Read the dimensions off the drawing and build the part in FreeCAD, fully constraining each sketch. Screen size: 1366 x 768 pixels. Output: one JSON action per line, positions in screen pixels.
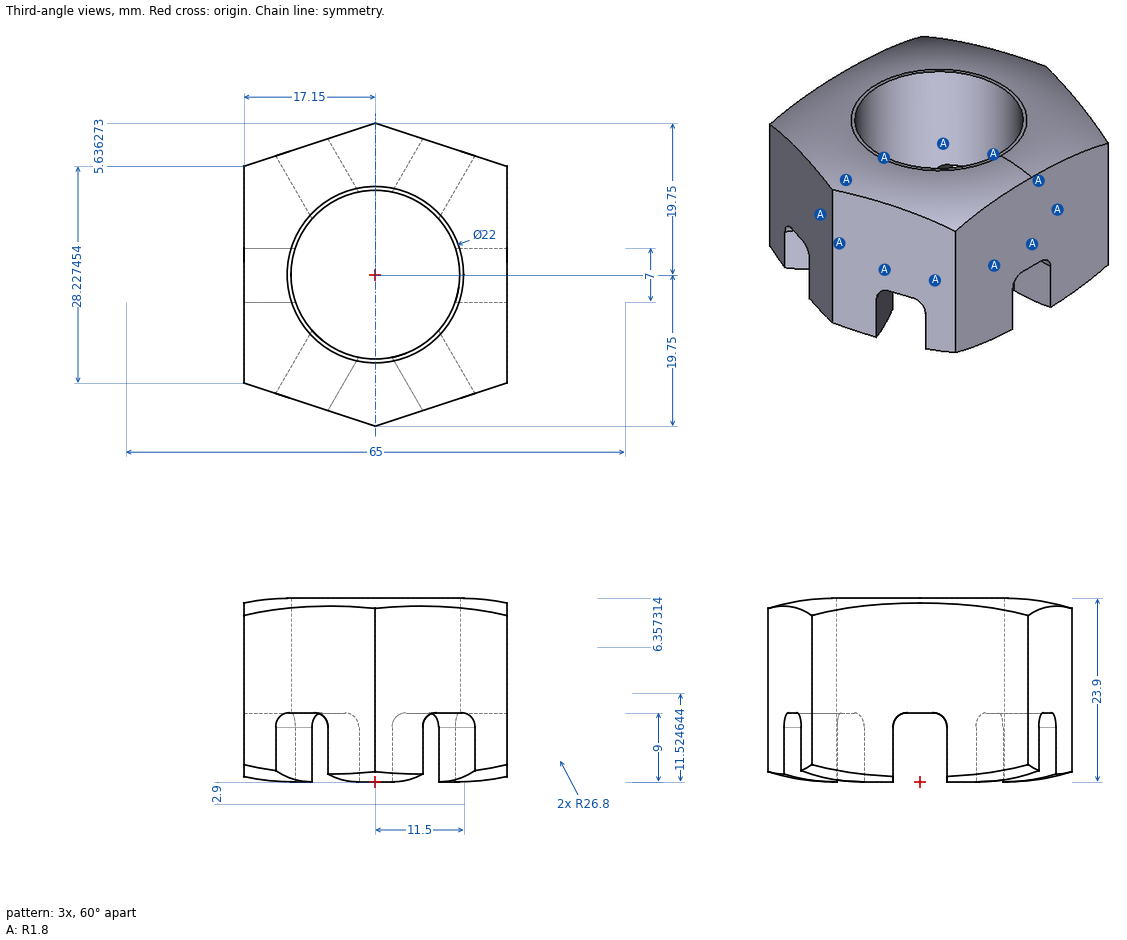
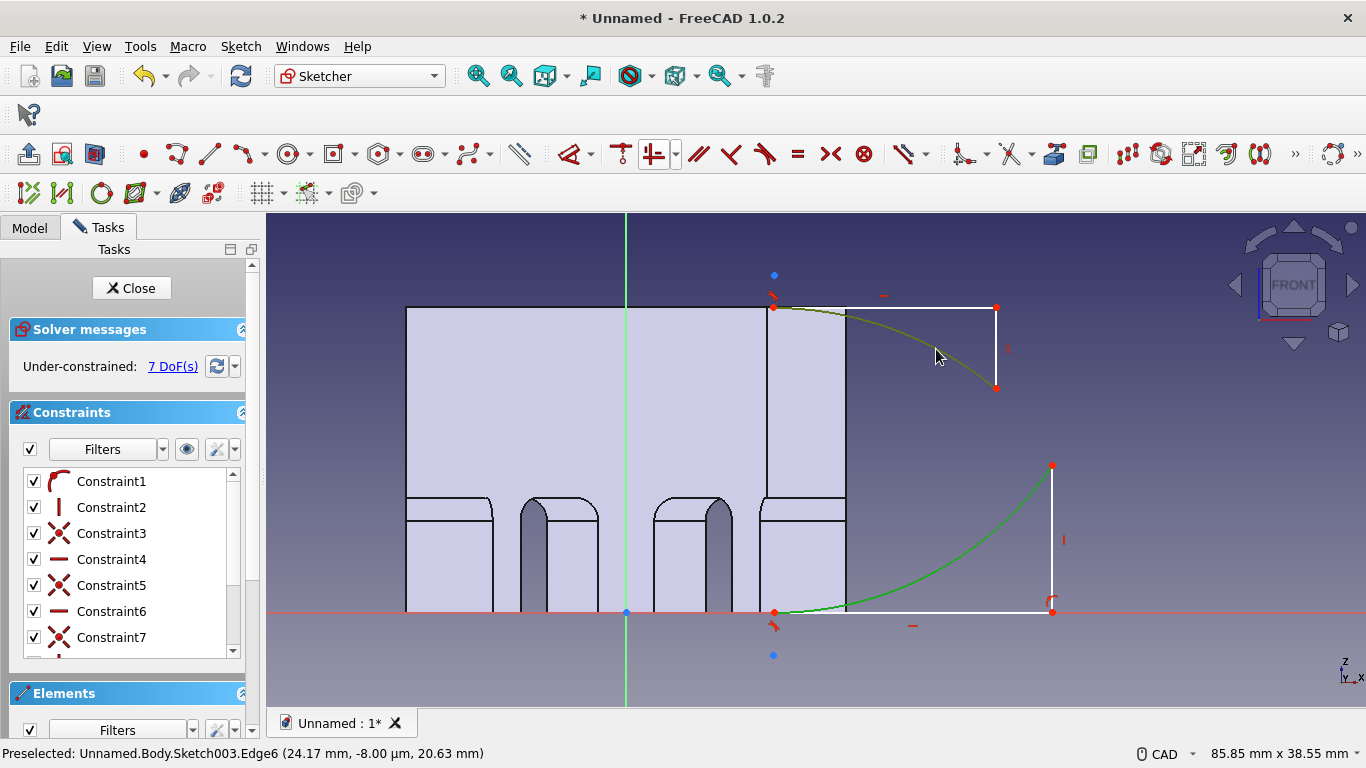
{"action": "left_click", "coordinate": [798, 154]}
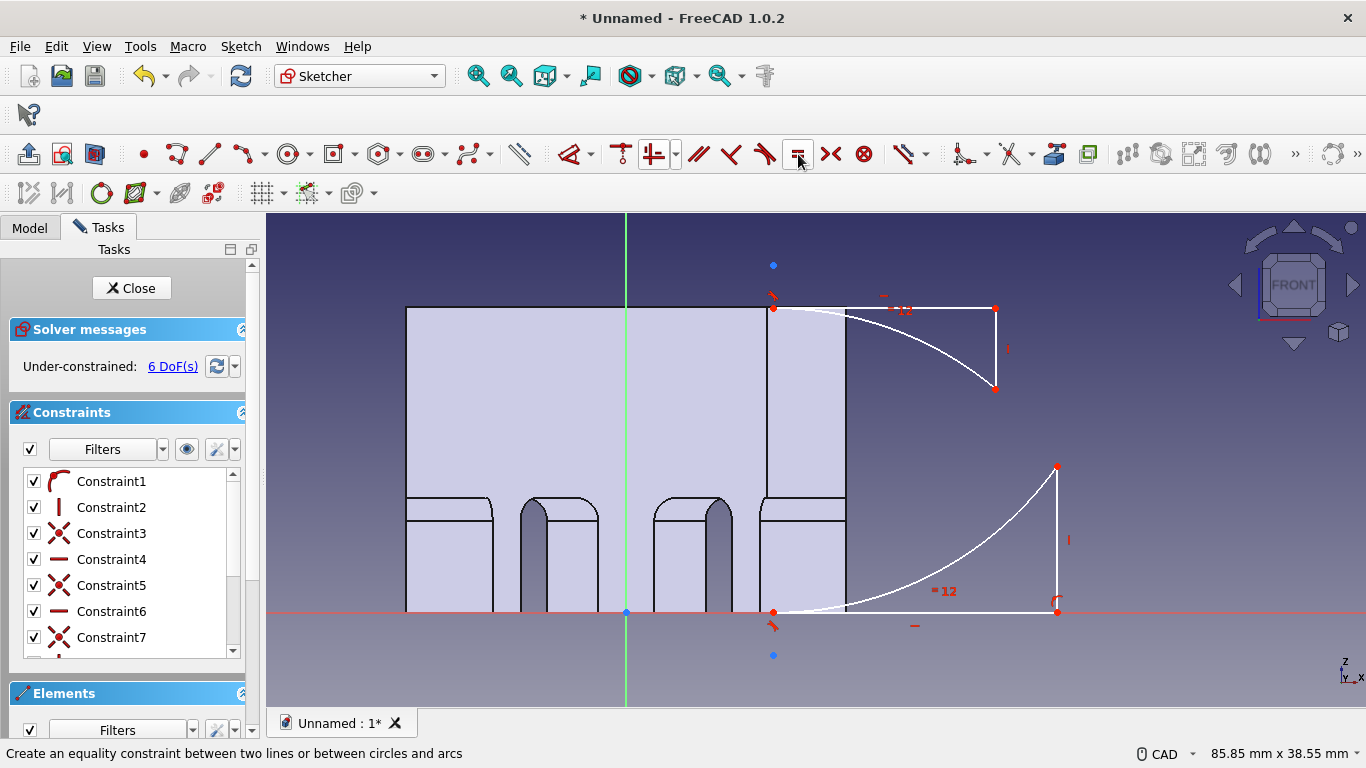
{"action": "left_click", "coordinate": [568, 154]}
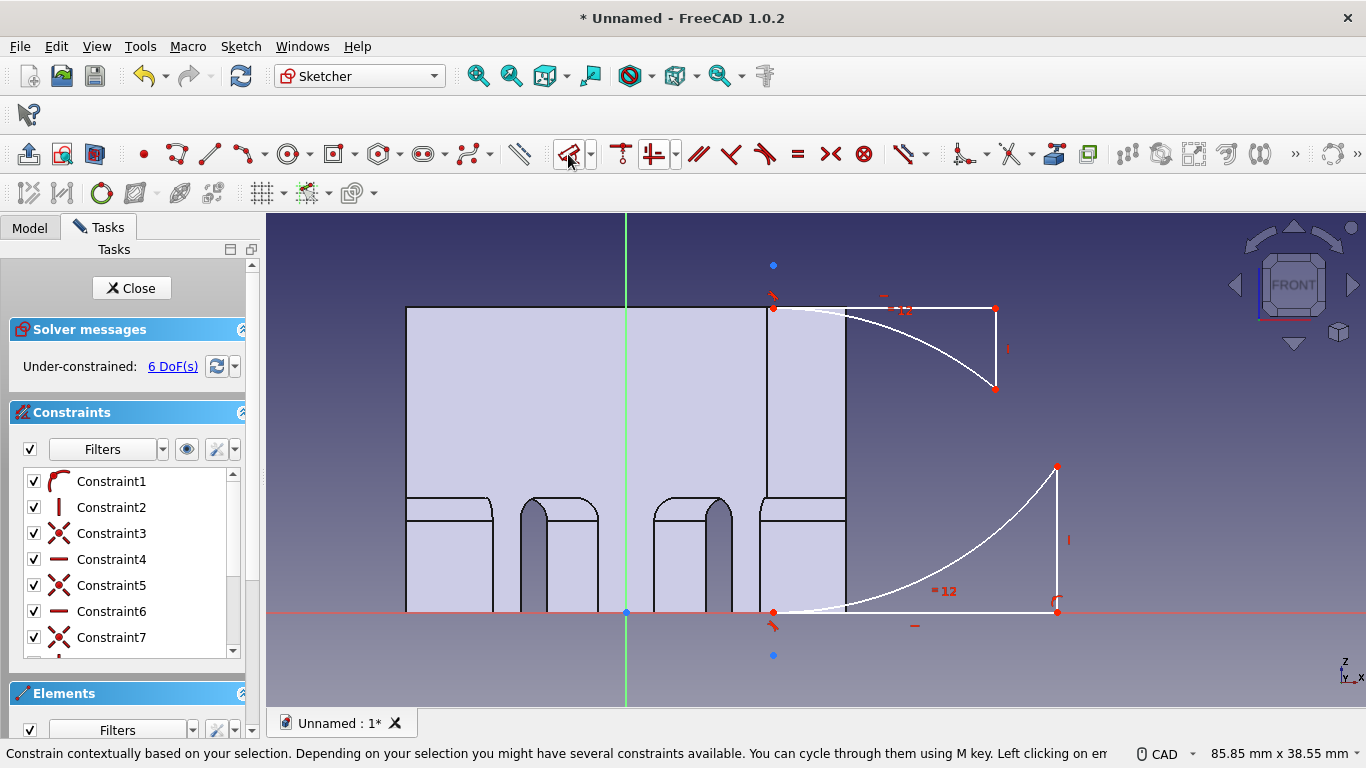
{"action": "left_click", "coordinate": [872, 599]}
{"action": "left_click", "coordinate": [881, 630]}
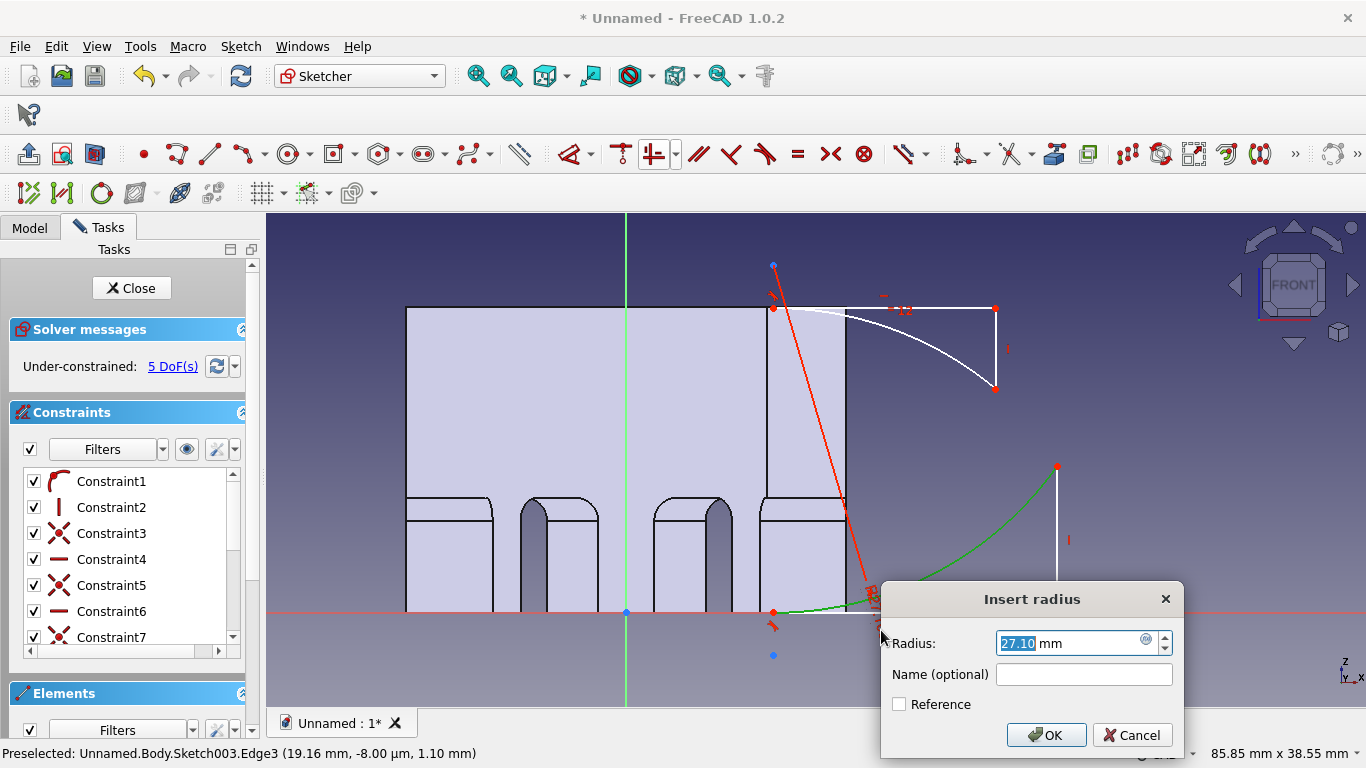
{"action": "type", "text": "26.8"}
{"action": "key", "text": "Return"}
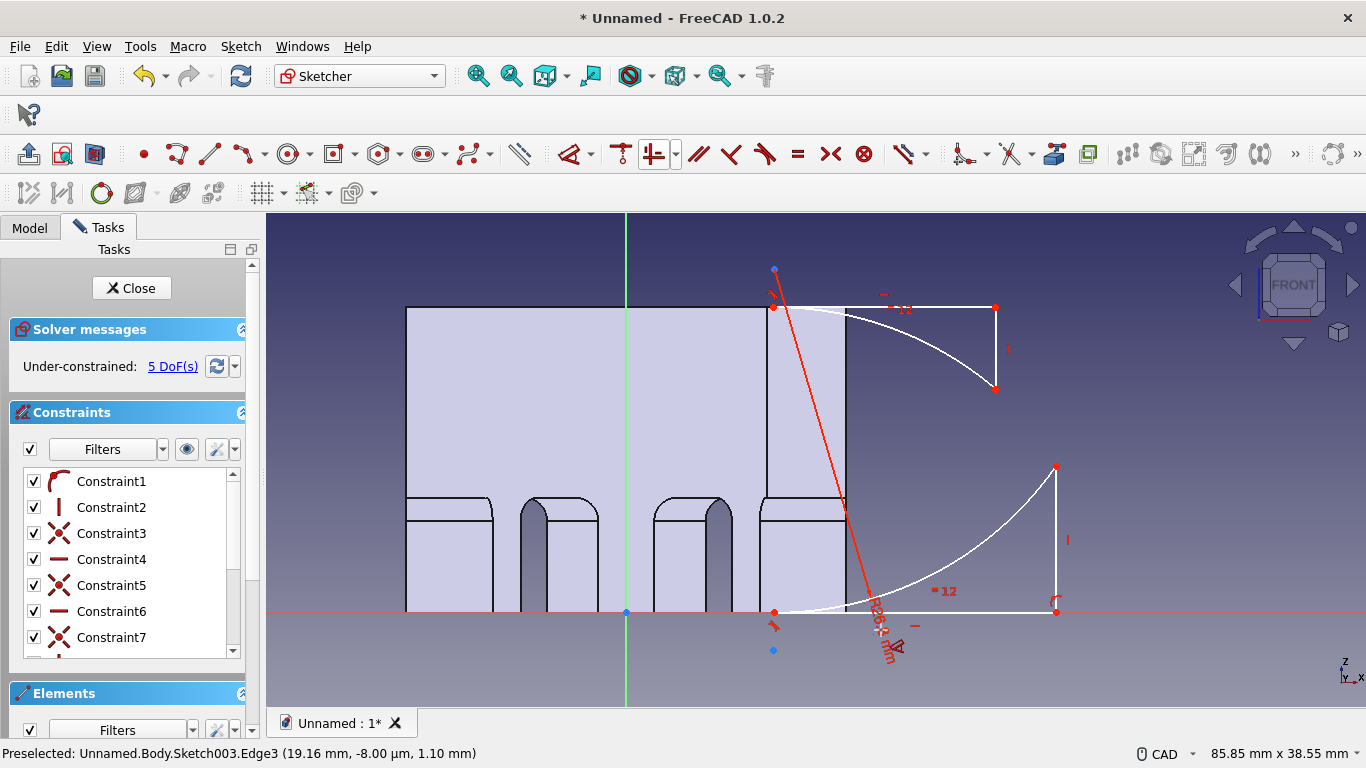
{"action": "left_click", "coordinate": [773, 650]}
{"action": "left_click", "coordinate": [592, 632]}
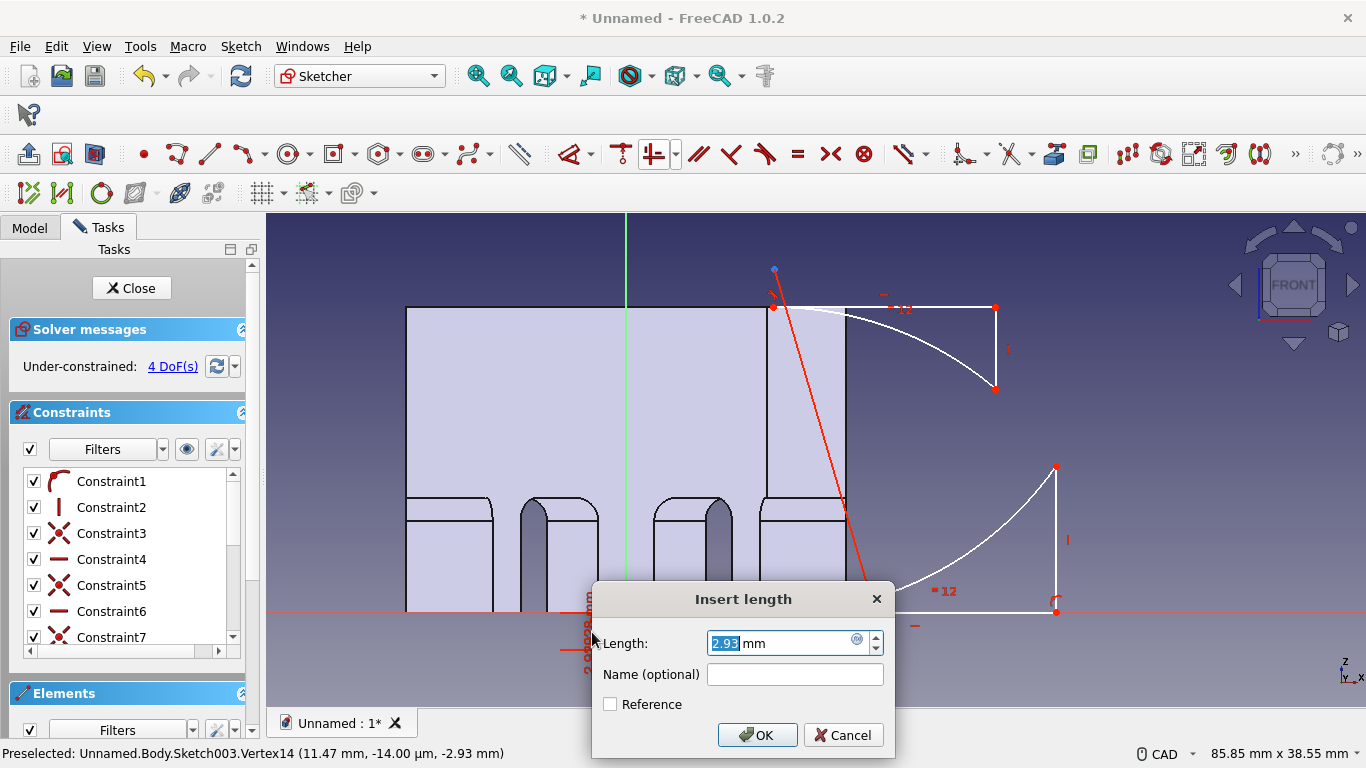
{"action": "type", "text": "2.9"}
{"action": "key", "text": "Return"}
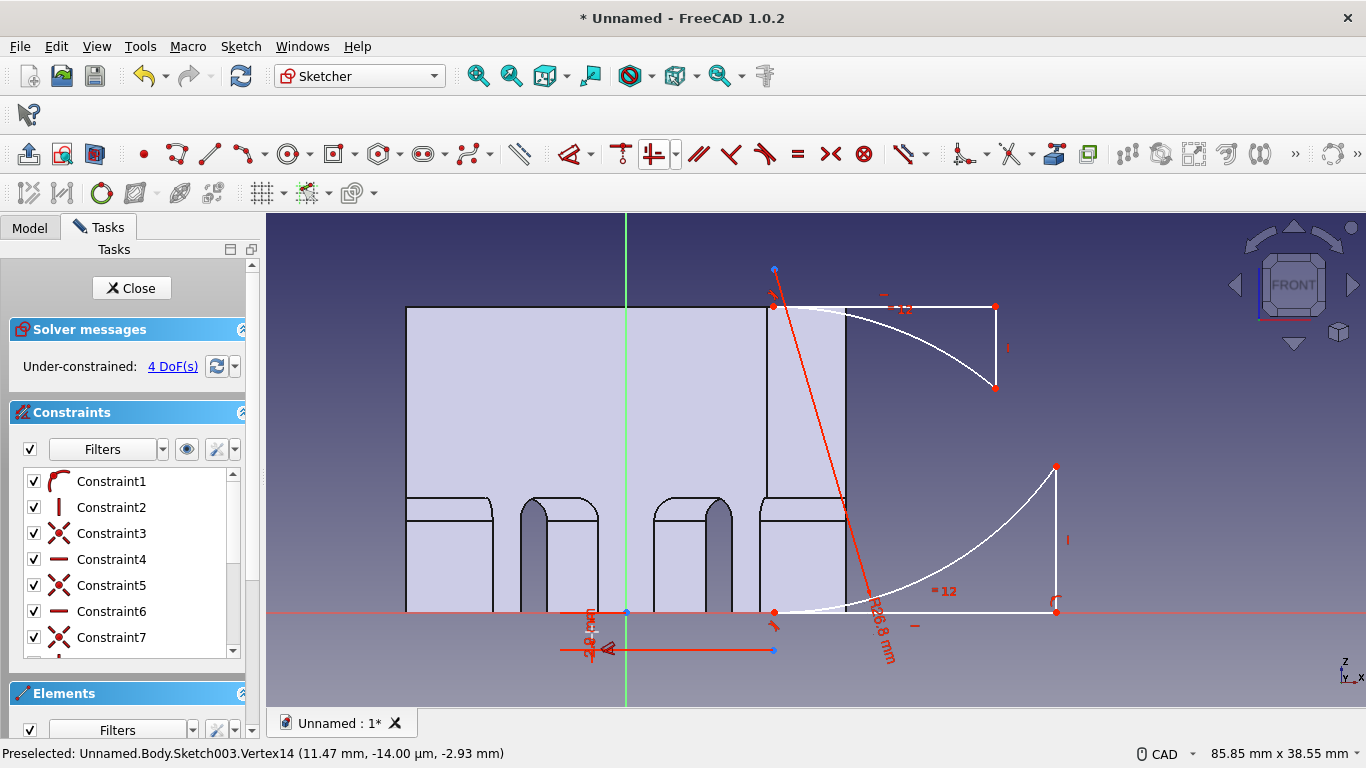
{"action": "left_click", "coordinate": [775, 613]}
{"action": "left_click", "coordinate": [700, 647]}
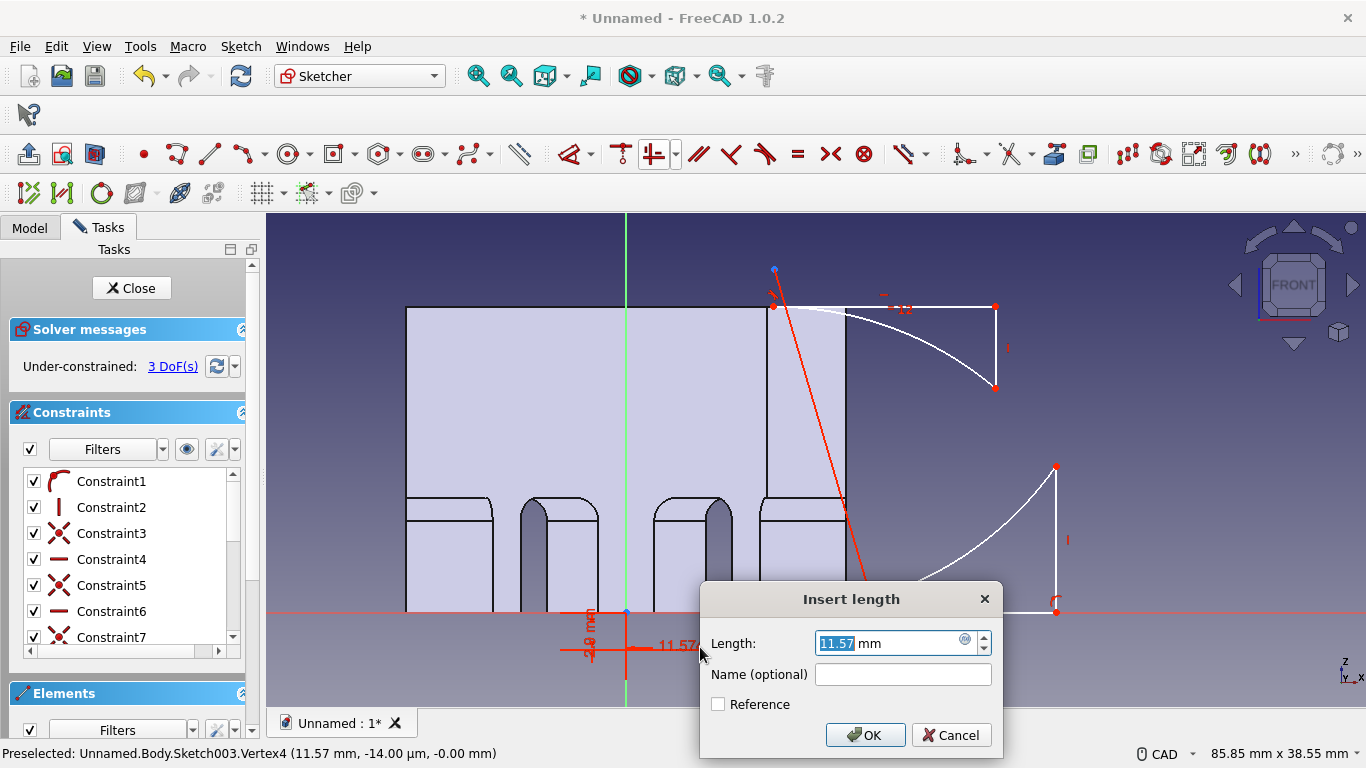
{"action": "type", "text": "11.5"}
{"action": "key", "text": "Return"}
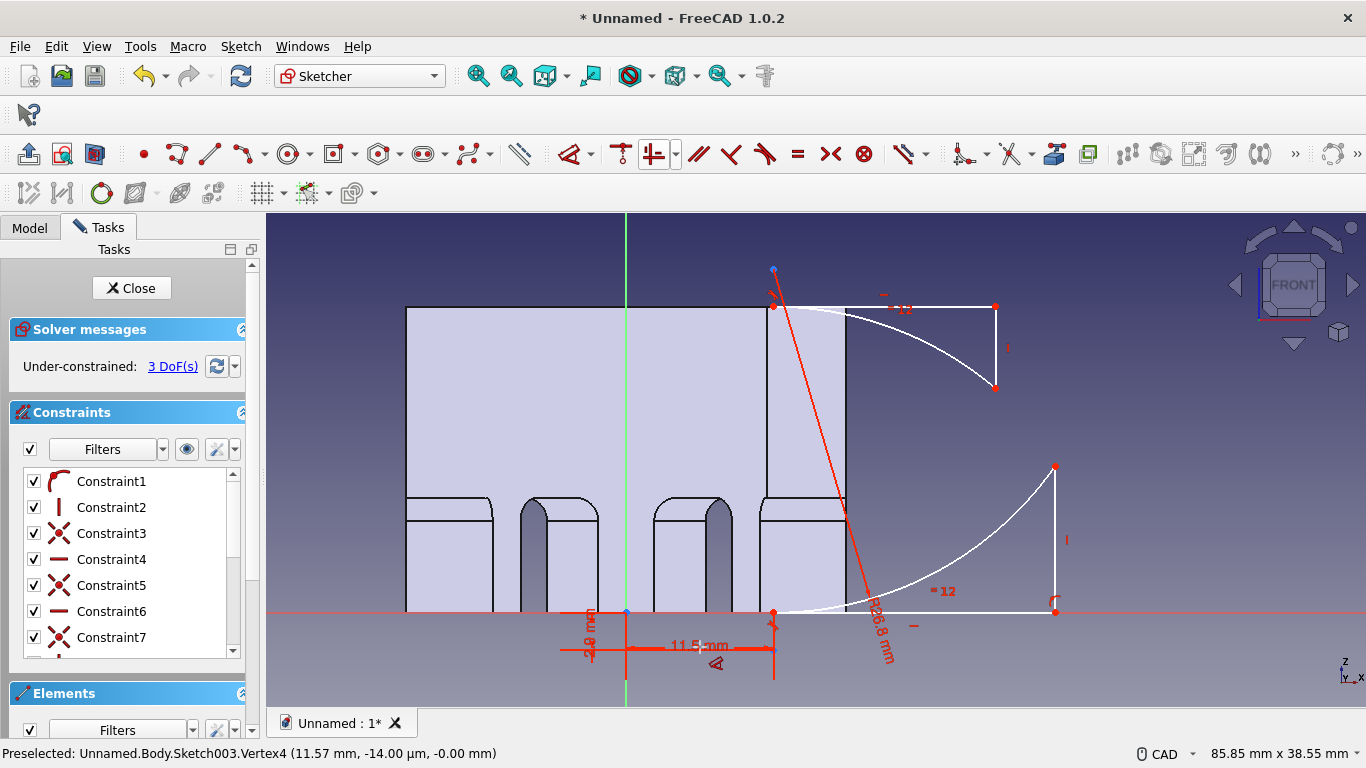
{"action": "left_click", "coordinate": [773, 307]}
{"action": "left_click", "coordinate": [700, 273]}